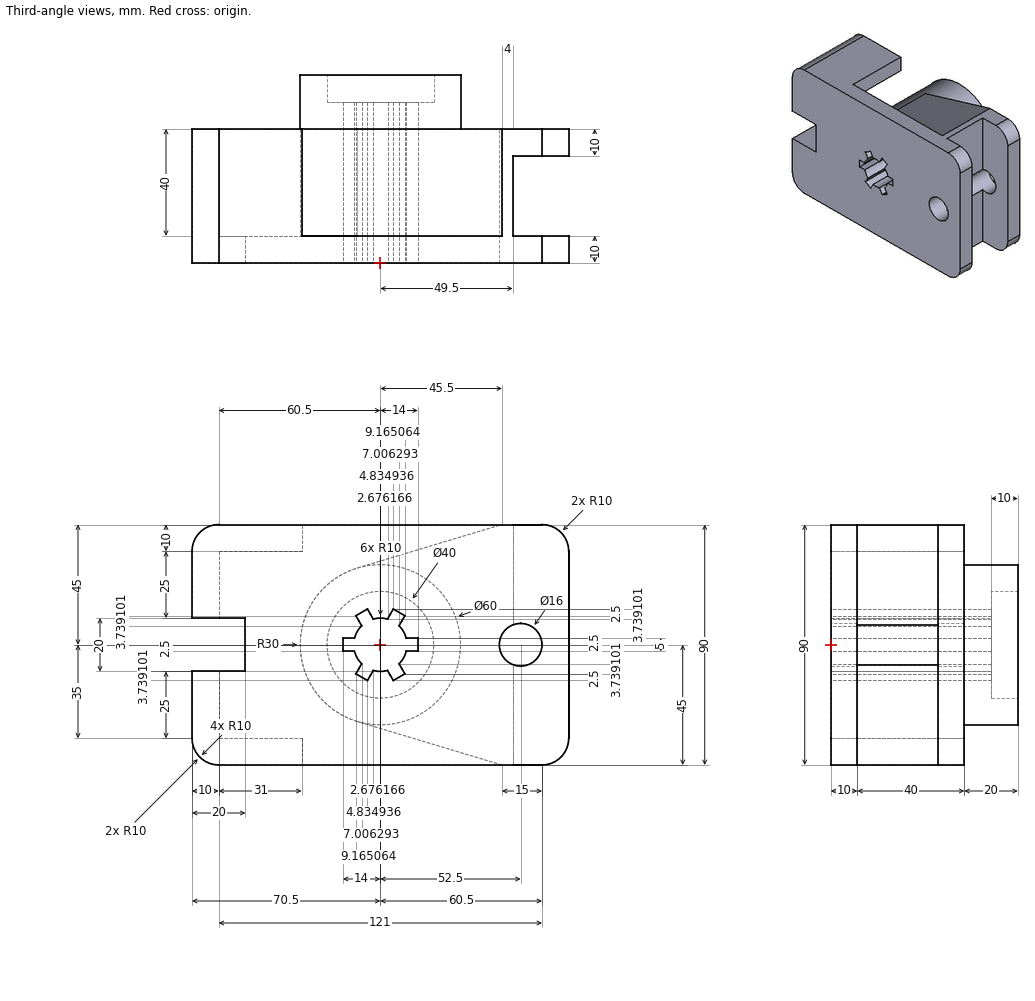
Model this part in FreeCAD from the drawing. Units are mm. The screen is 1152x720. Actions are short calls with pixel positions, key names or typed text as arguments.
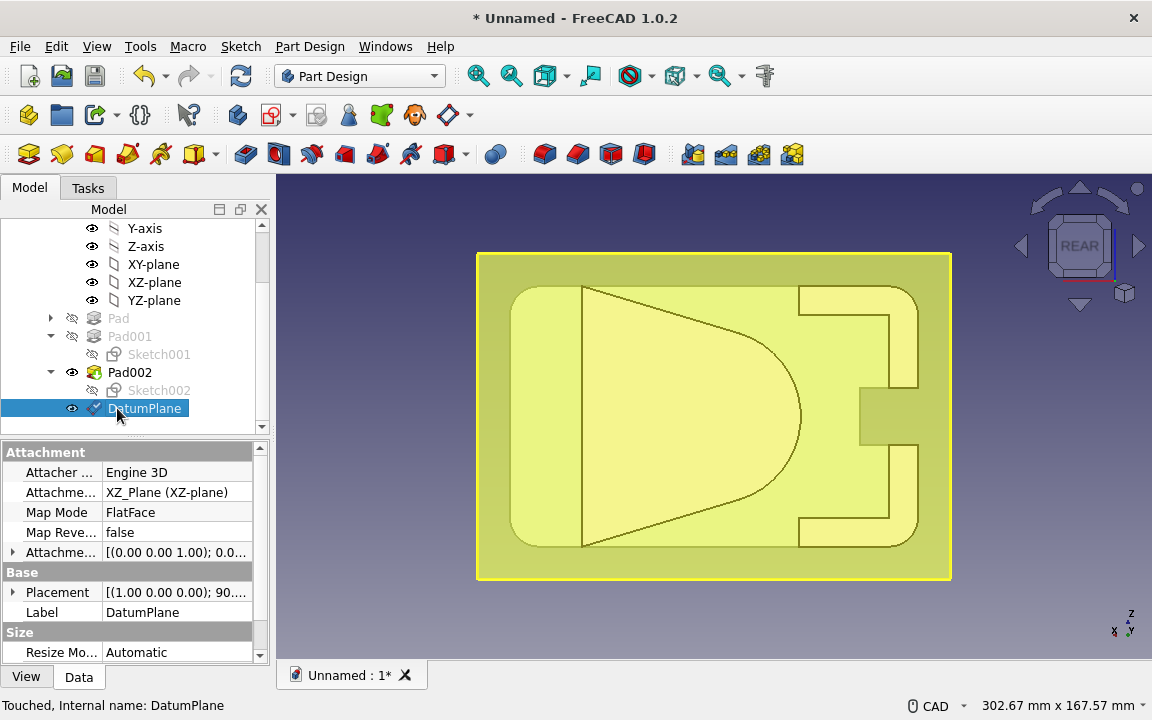
click(270, 116)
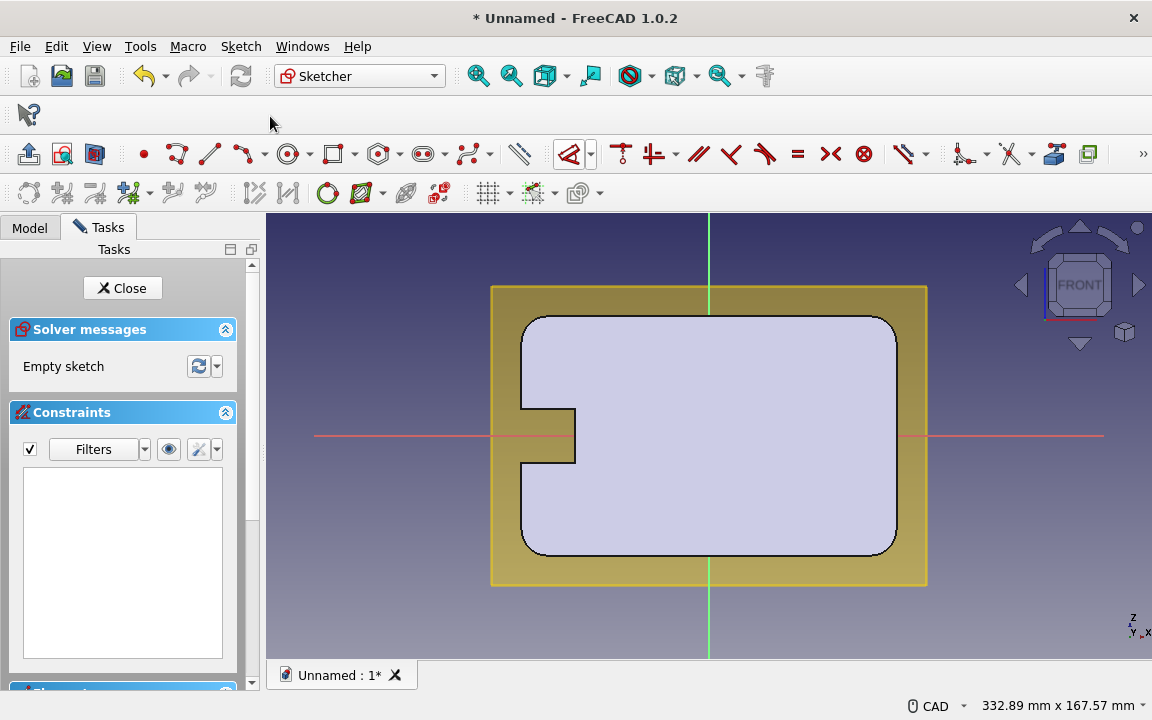
click(95, 154)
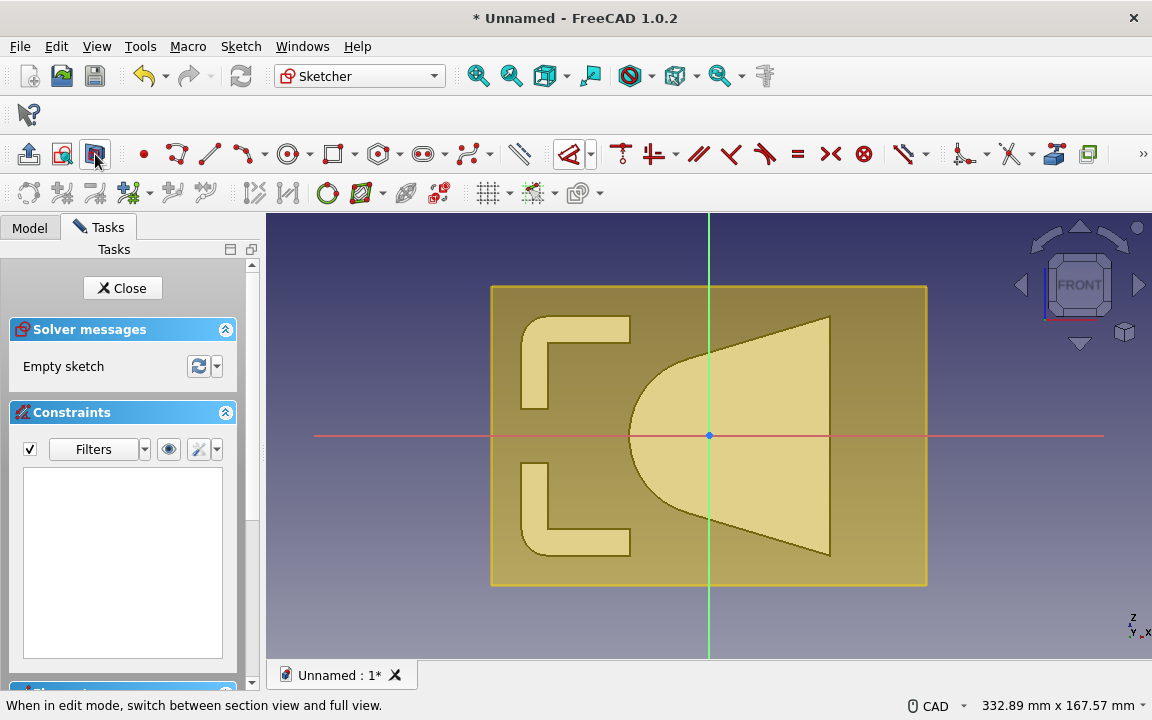
click(177, 154)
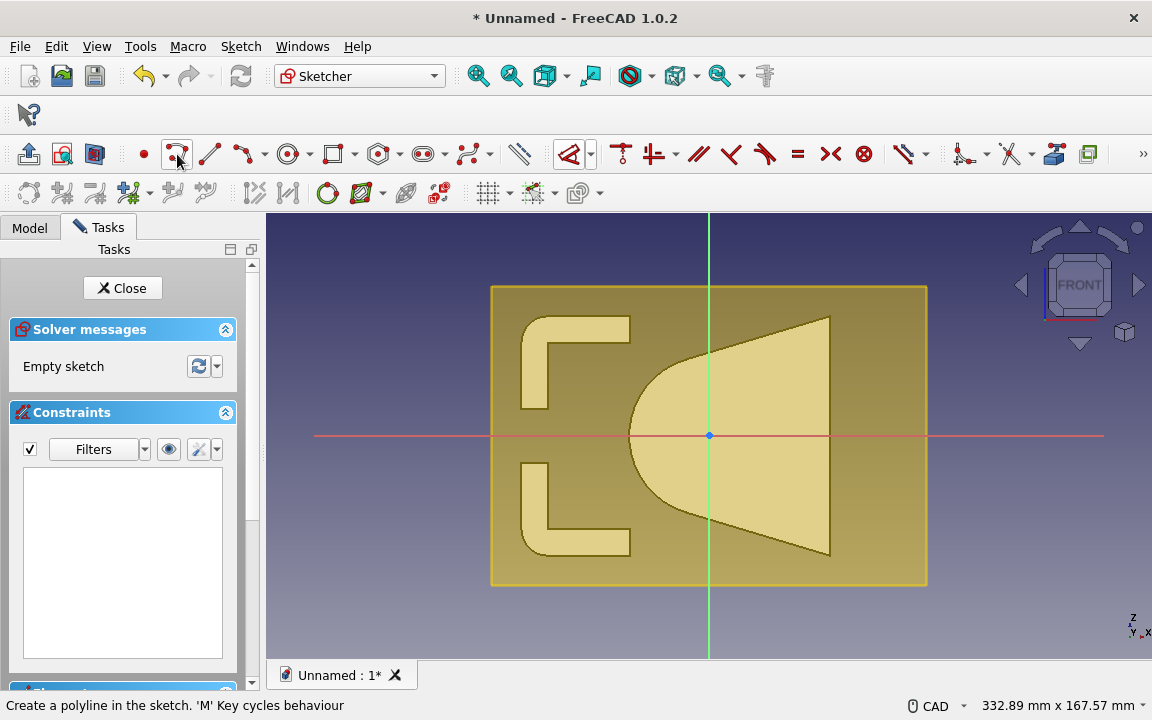
click(870, 556)
click(830, 556)
click(830, 316)
click(870, 316)
right_click(870, 316)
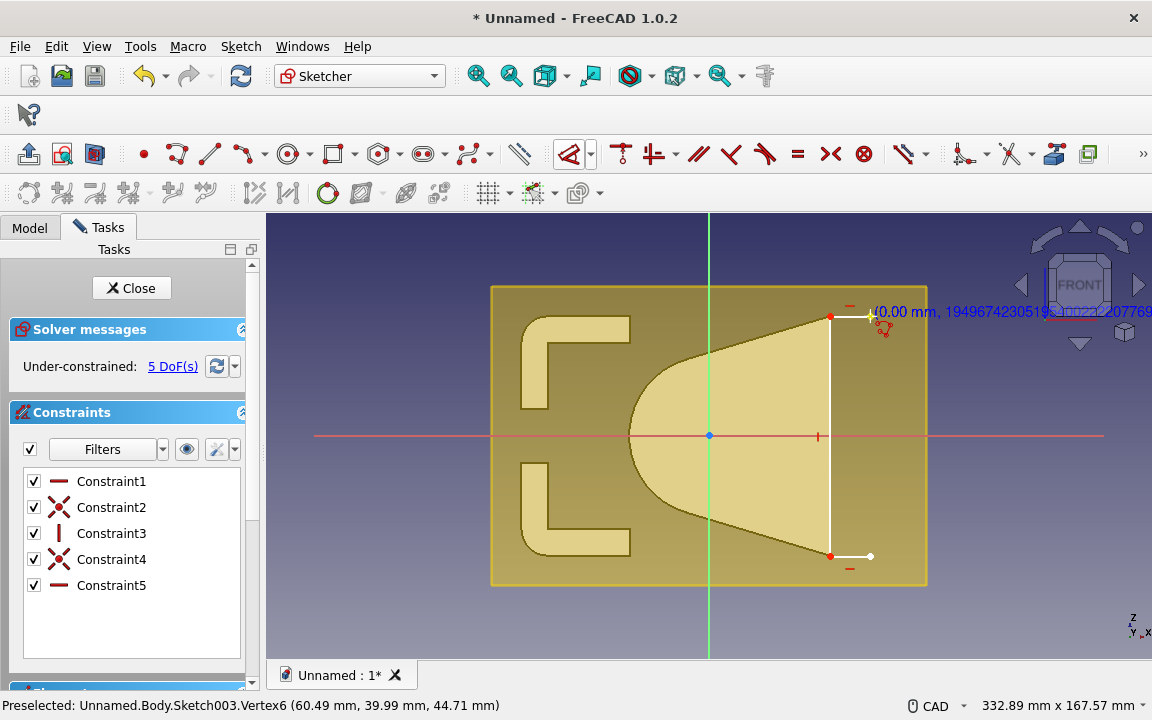
click(210, 154)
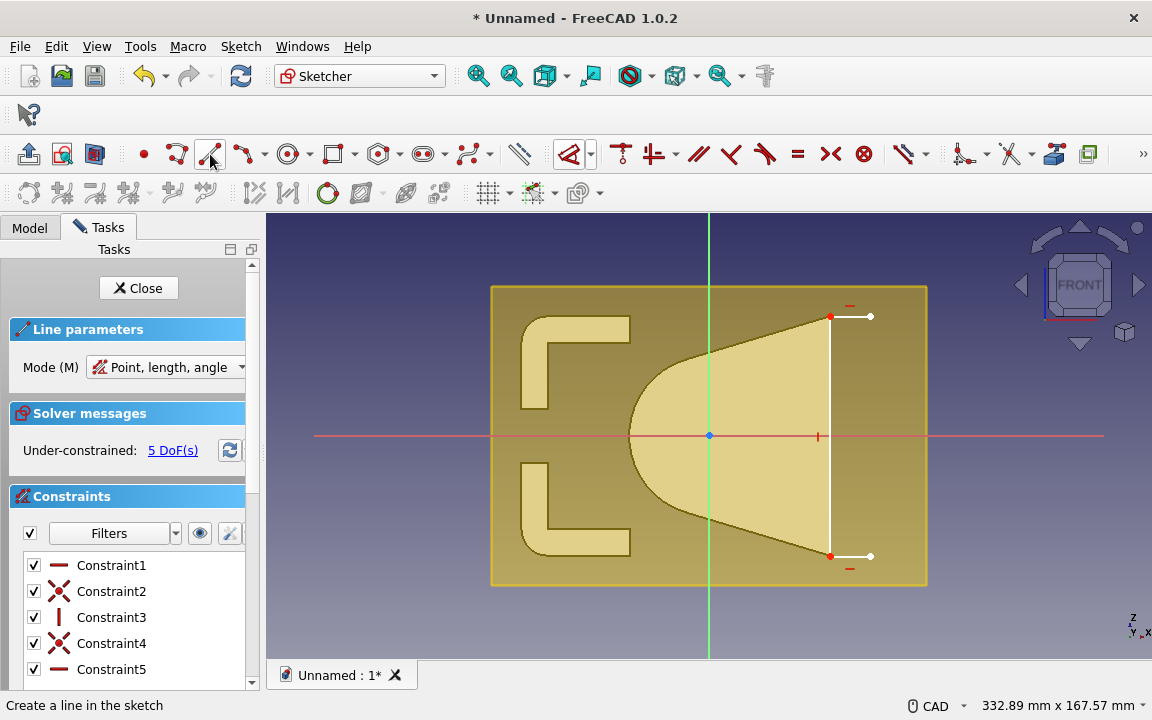
click(897, 343)
click(897, 529)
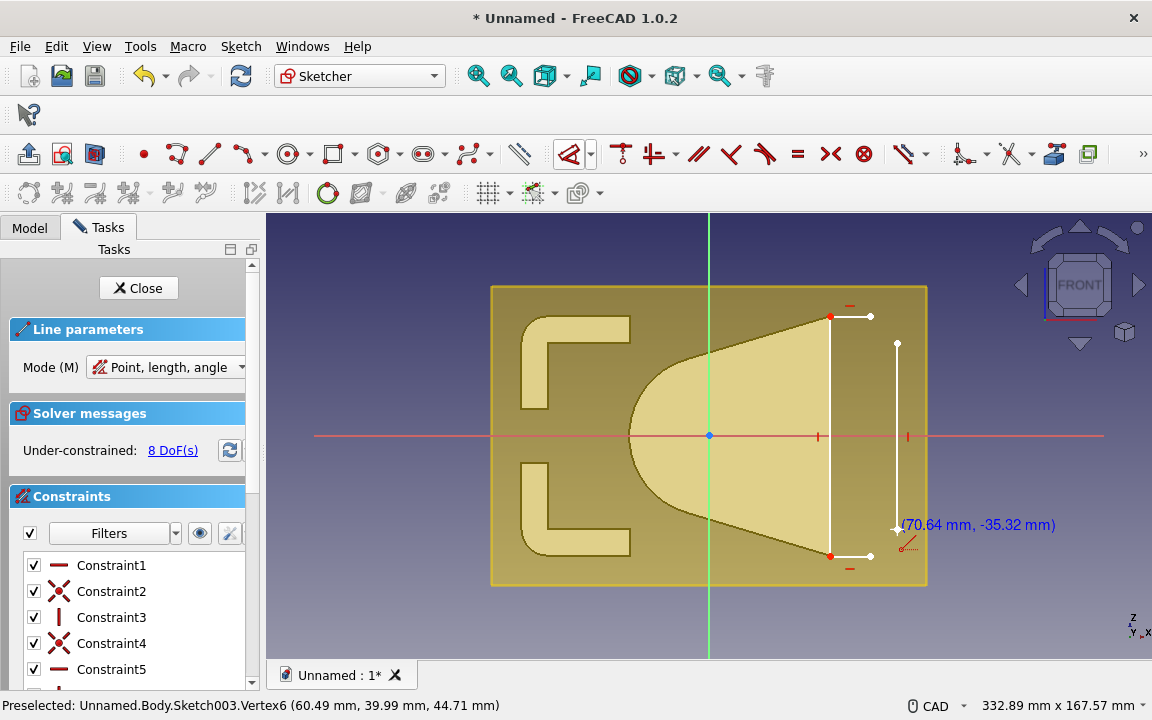
click(242, 154)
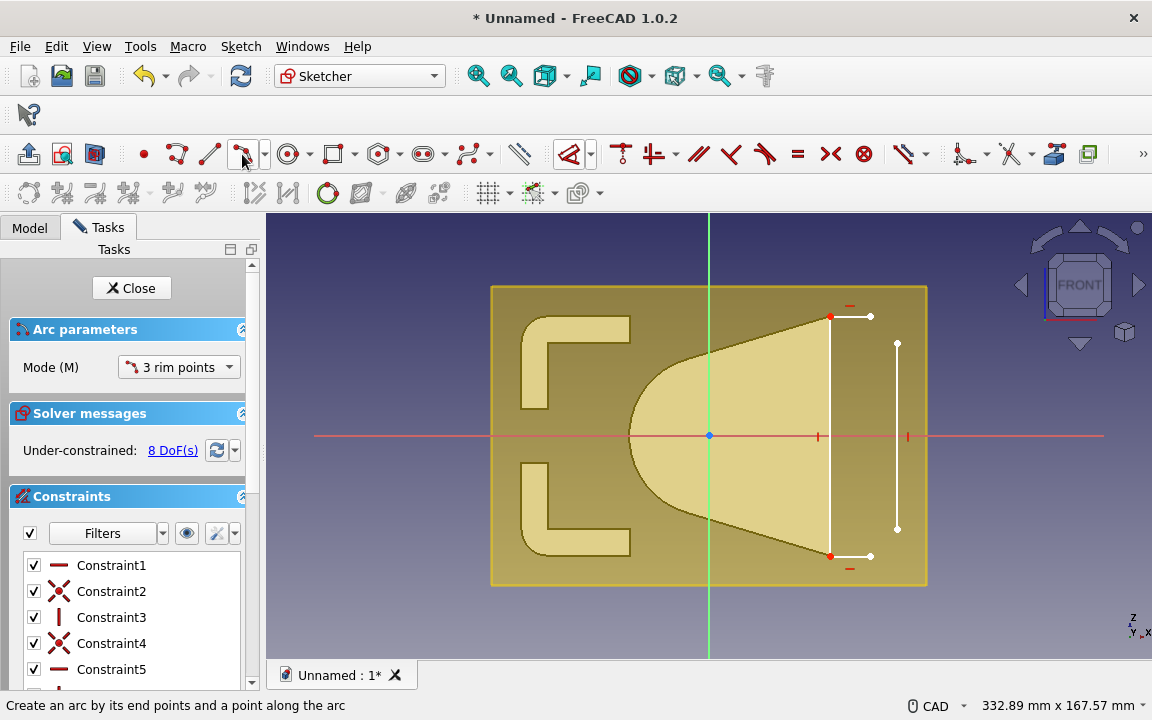
click(870, 317)
click(897, 344)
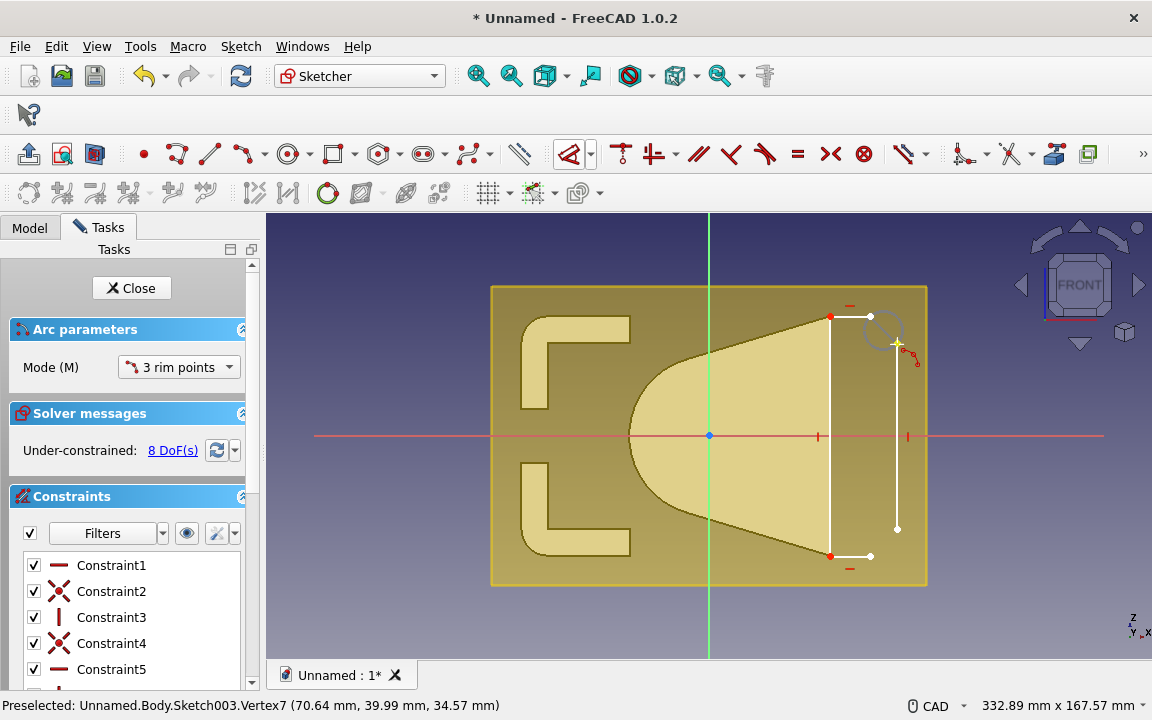
scroll(889, 324, up, 4)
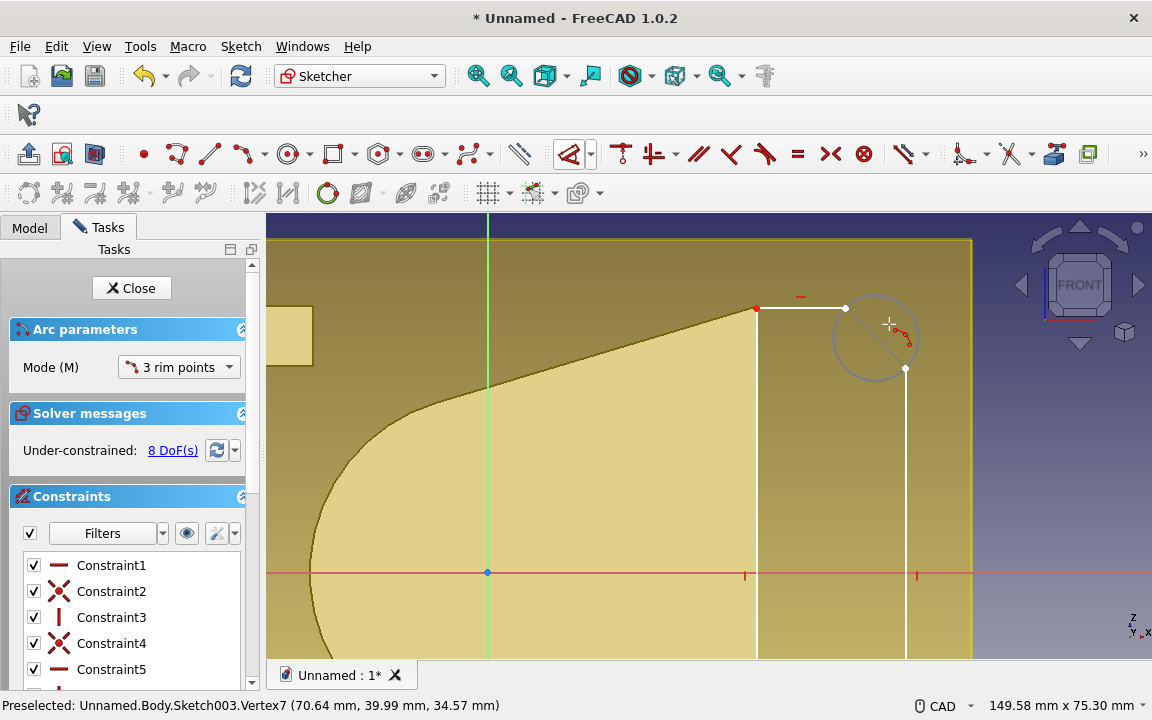
click(888, 324)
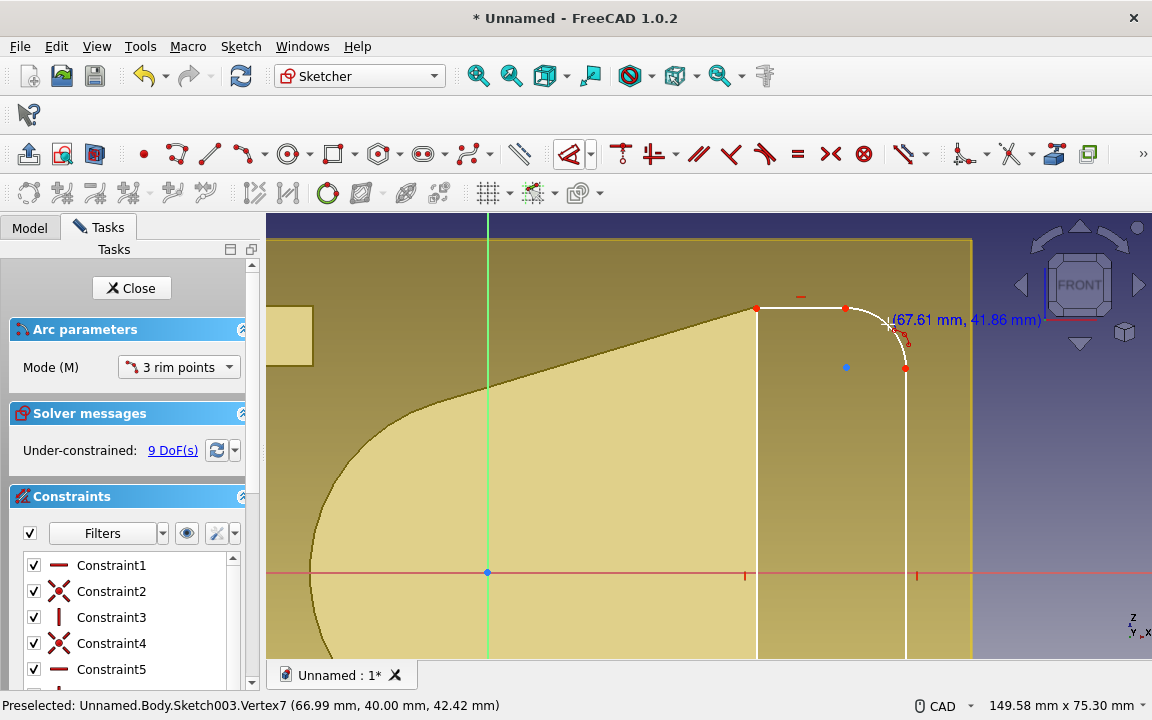
scroll(573, 269, down, 3)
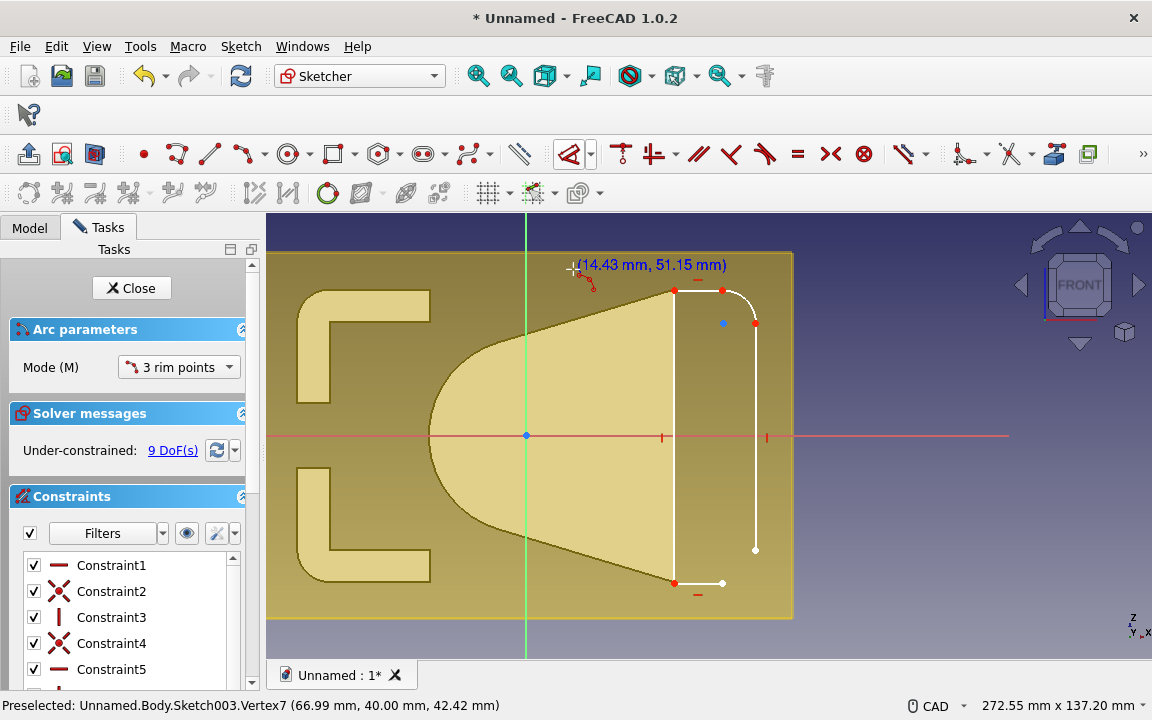
click(756, 551)
click(723, 584)